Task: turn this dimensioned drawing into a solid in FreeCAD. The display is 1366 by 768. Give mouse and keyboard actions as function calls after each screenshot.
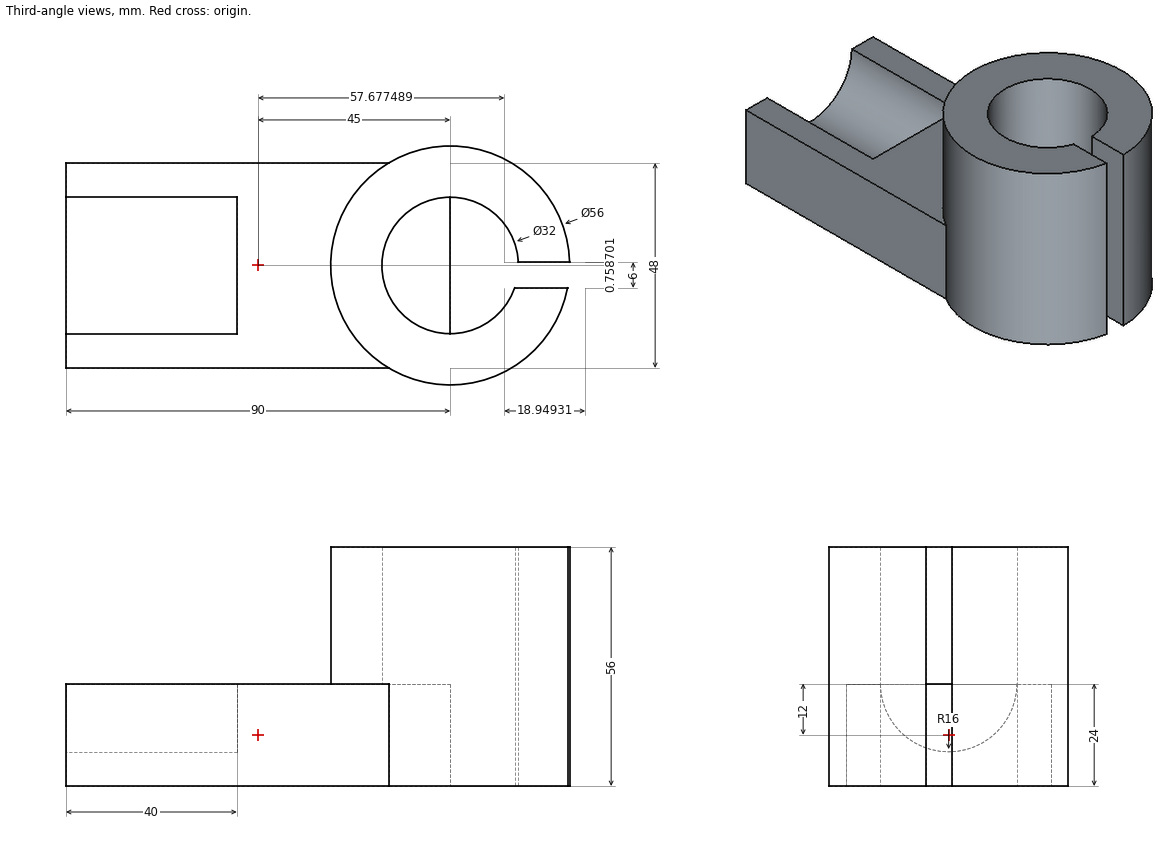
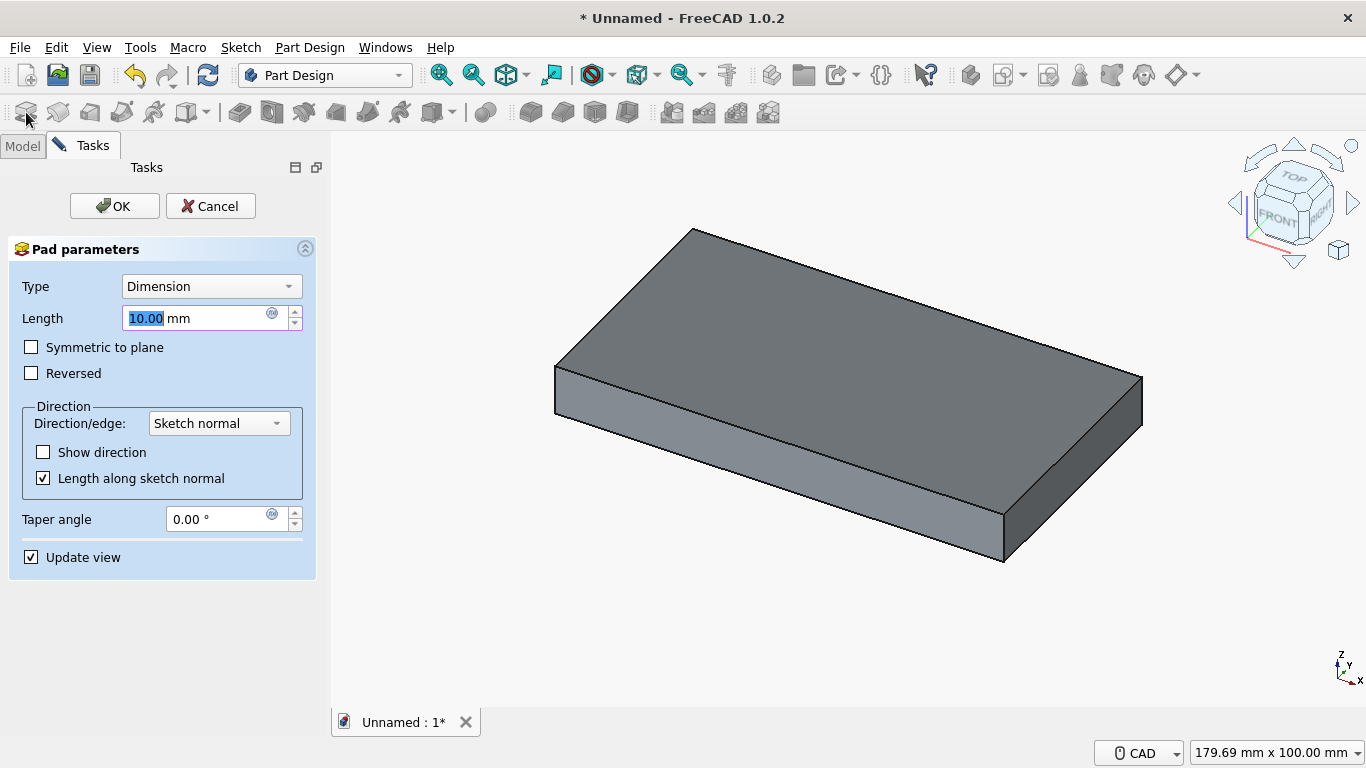
text(24)
key(Tab)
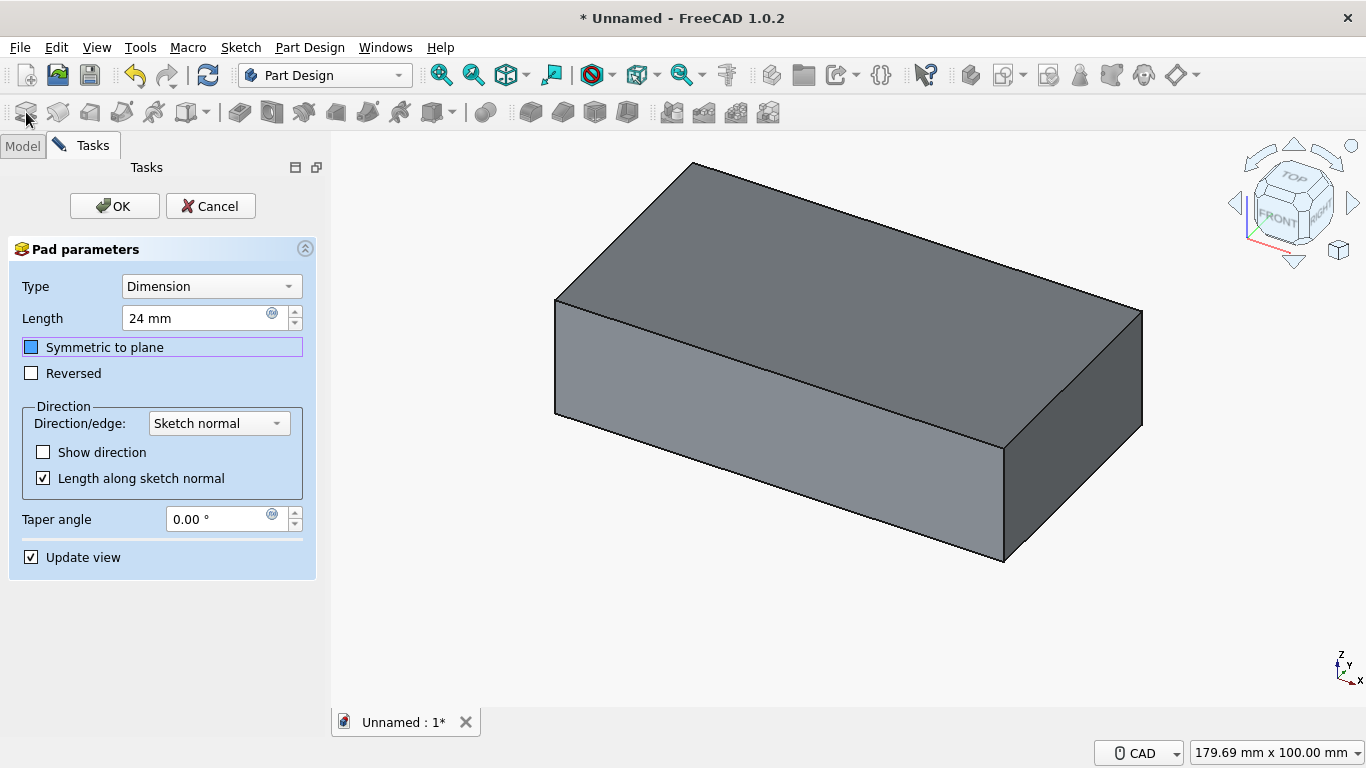
click(30, 347)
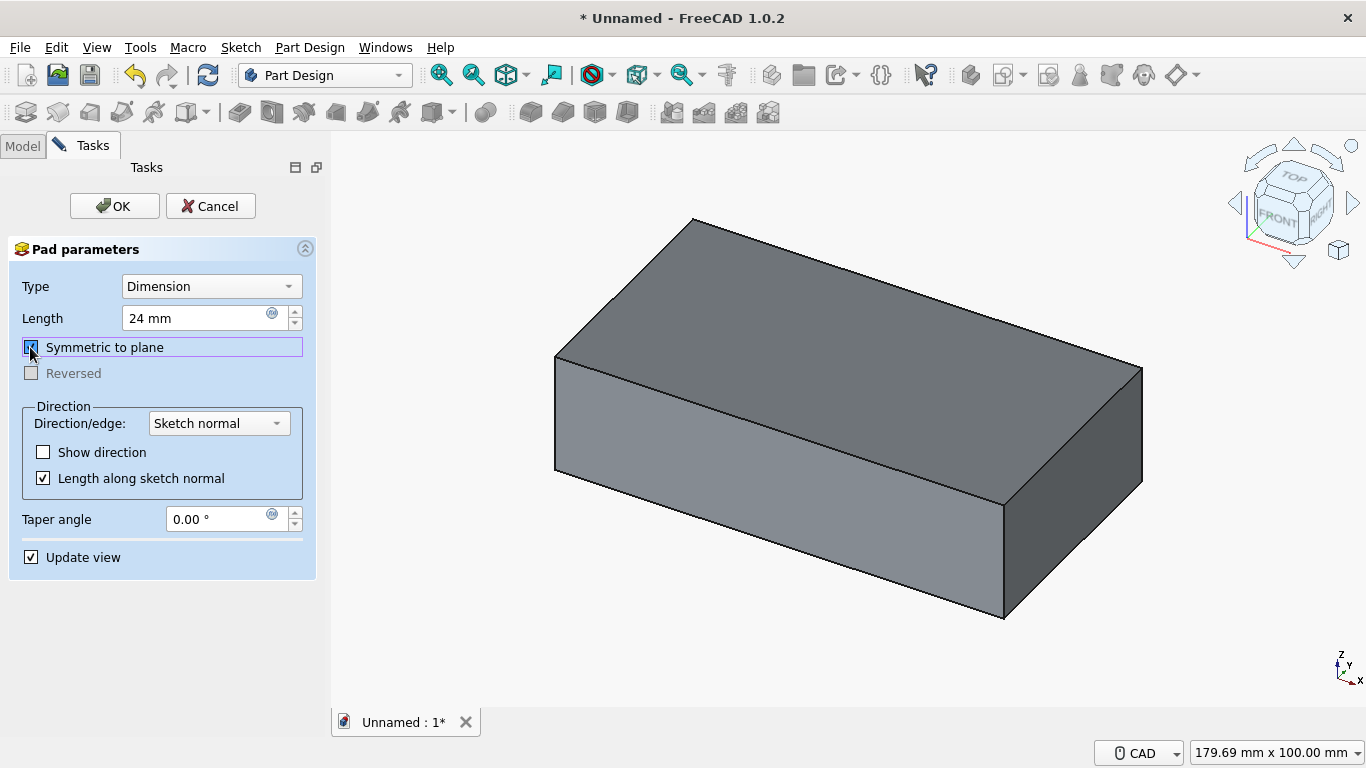
click(115, 206)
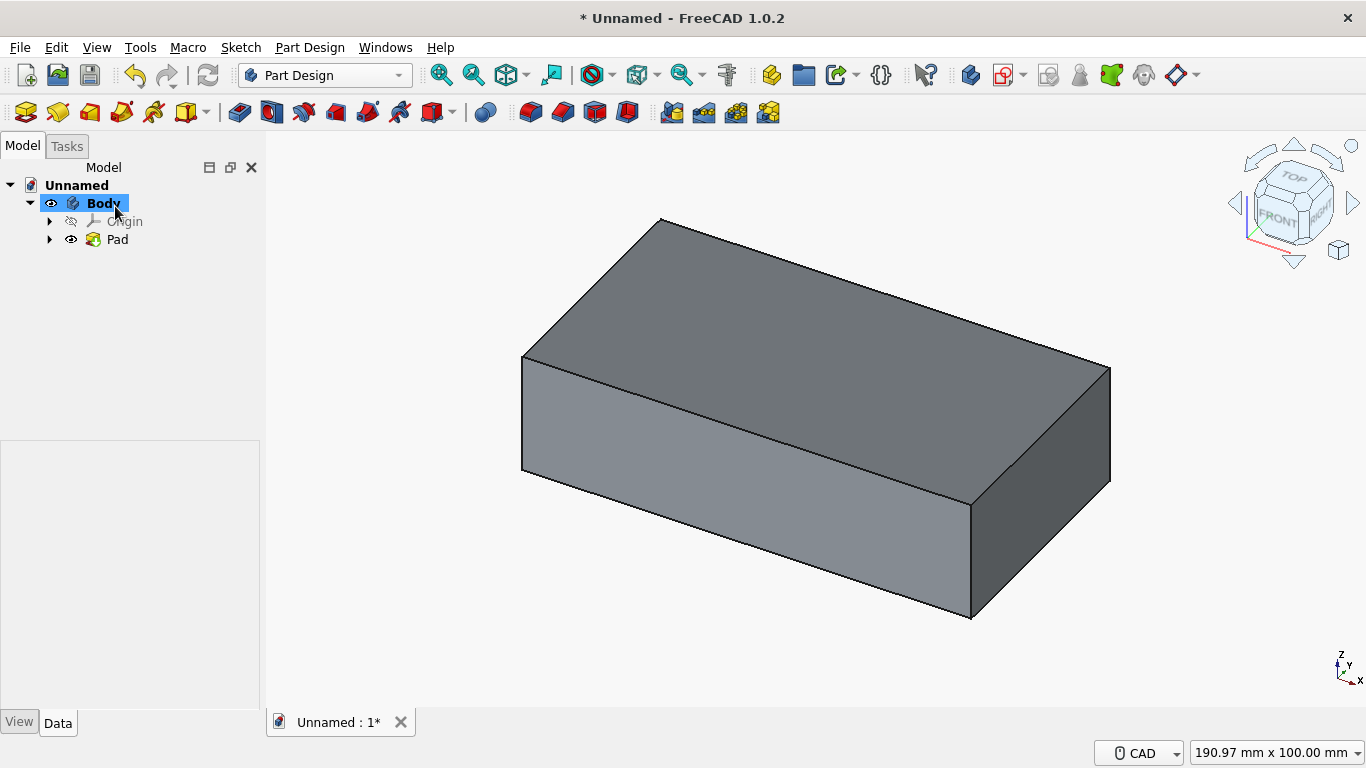
key(6)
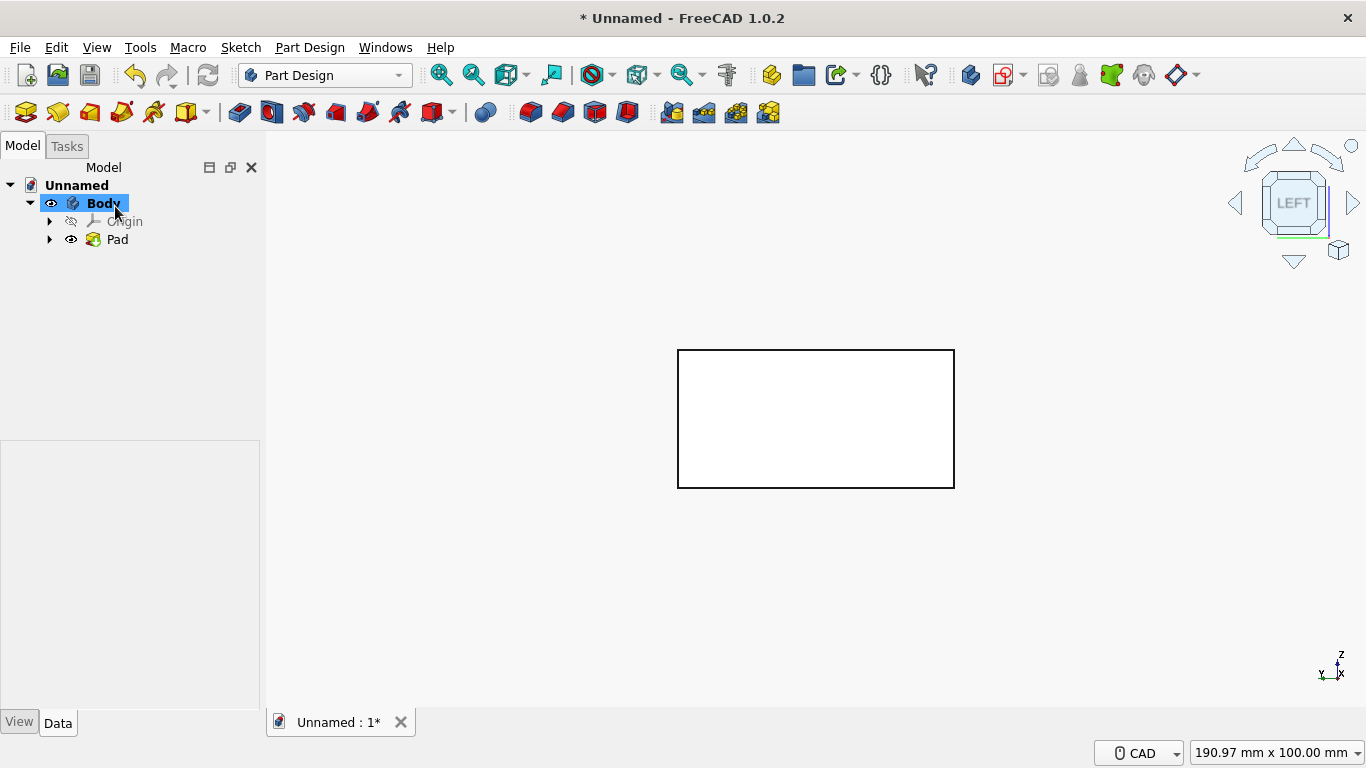
key(v)
key(f)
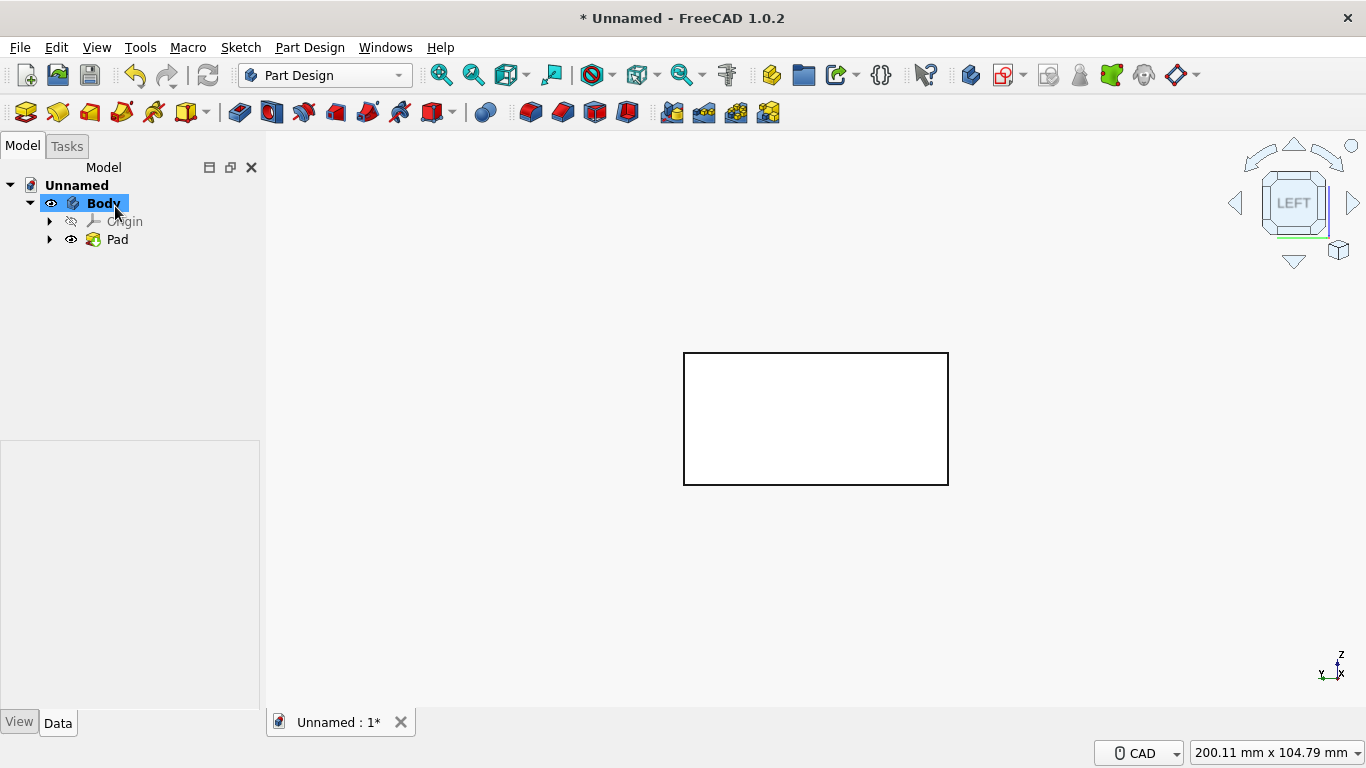
click(778, 418)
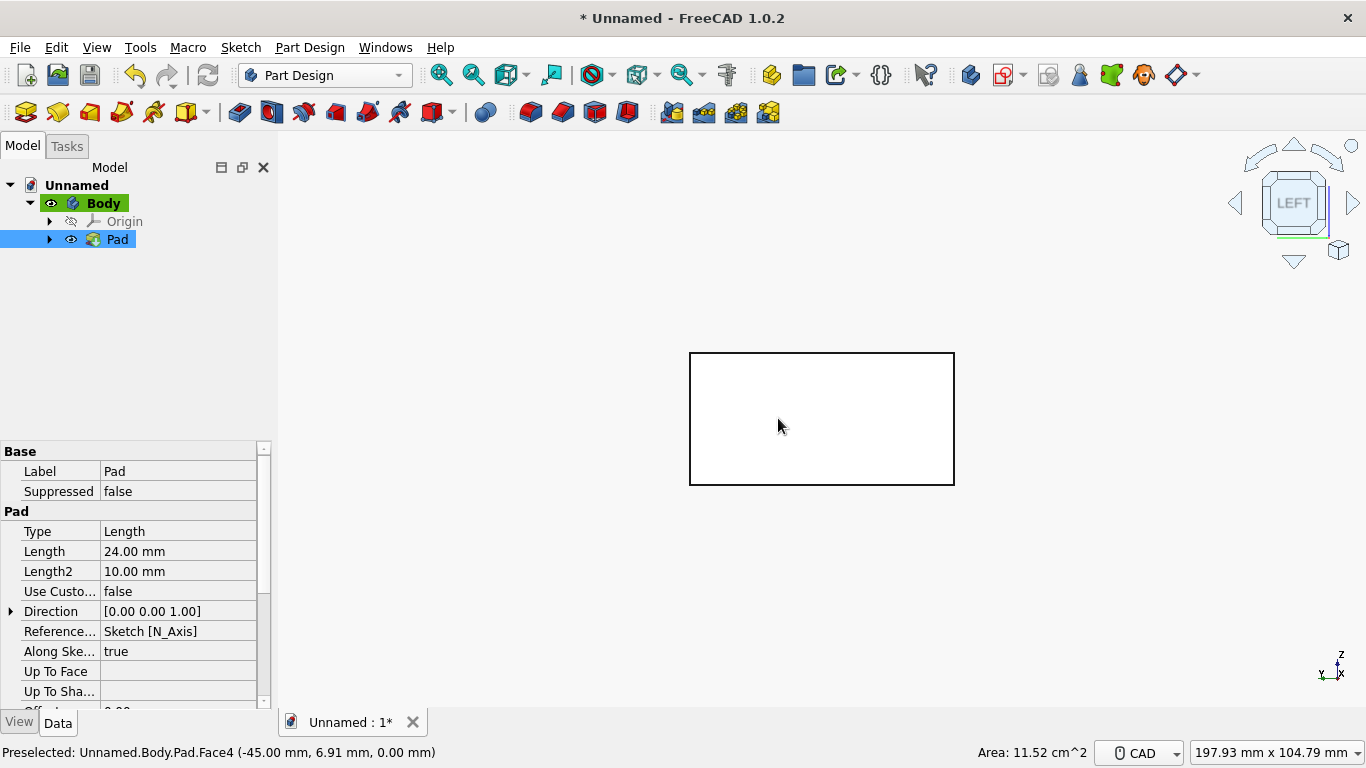
click(1004, 76)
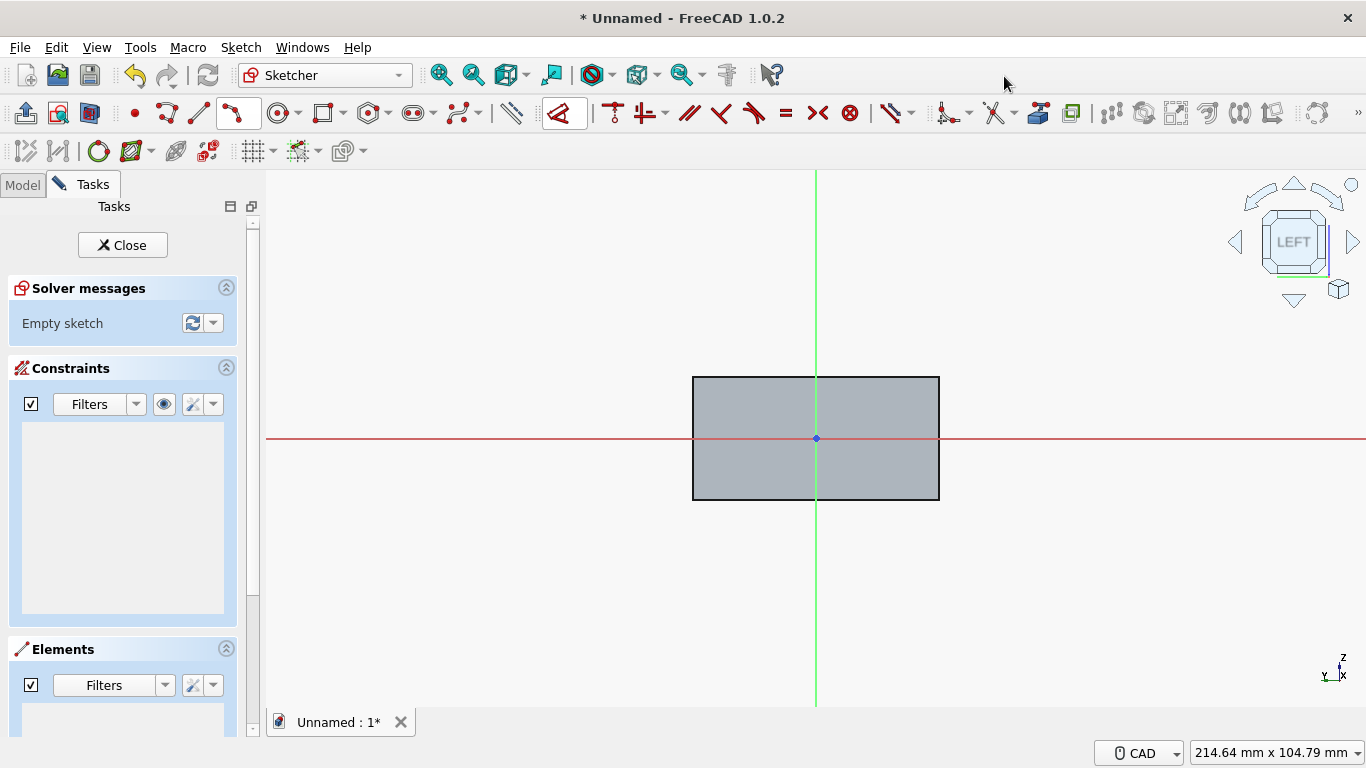
scroll(838, 411, up, 7)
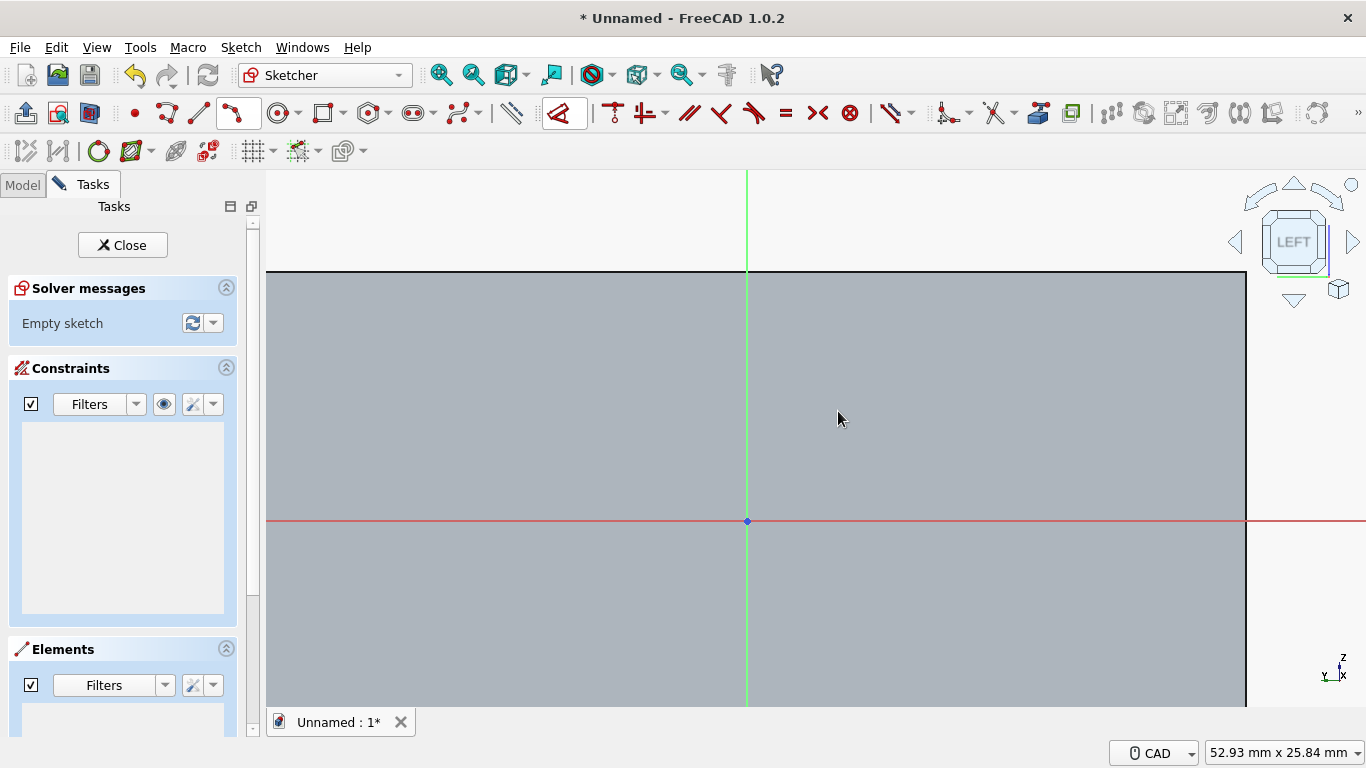
key(g)
key(l)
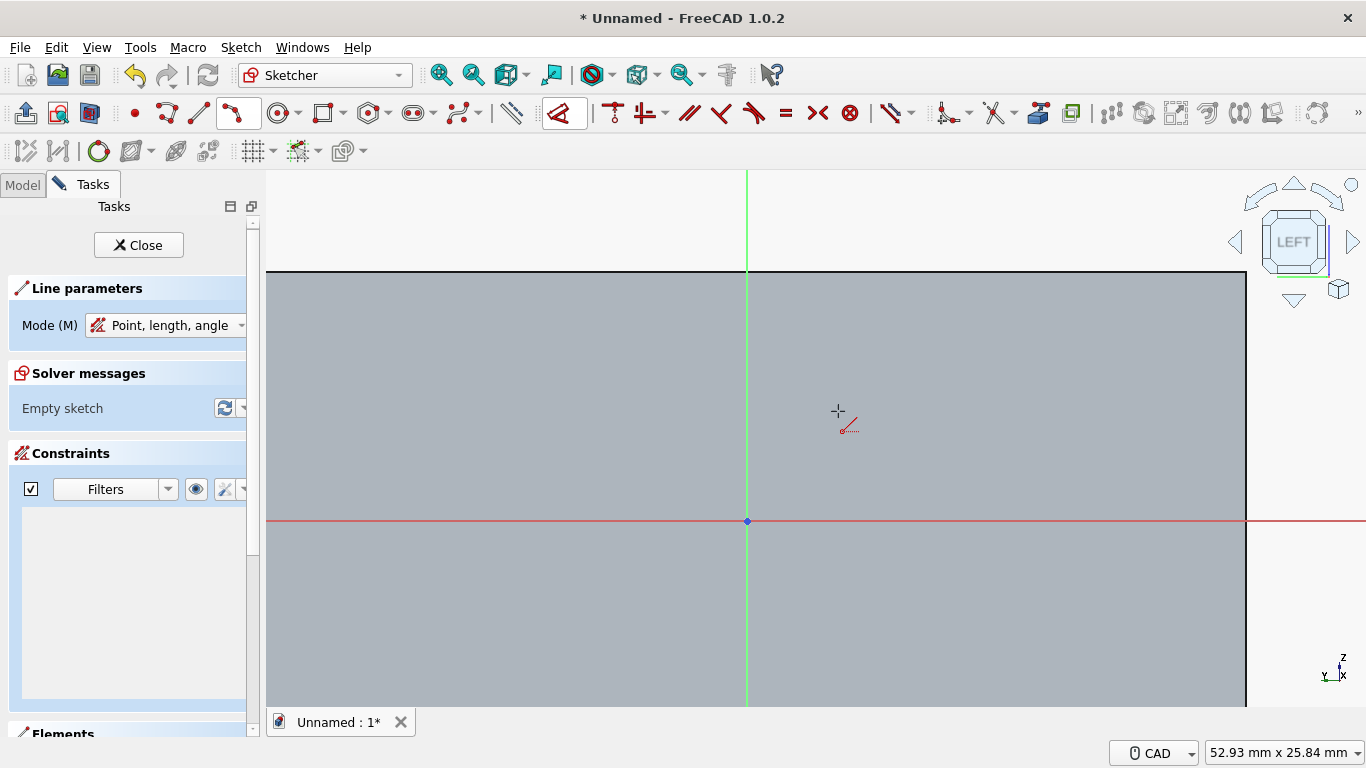
click(1080, 272)
click(415, 272)